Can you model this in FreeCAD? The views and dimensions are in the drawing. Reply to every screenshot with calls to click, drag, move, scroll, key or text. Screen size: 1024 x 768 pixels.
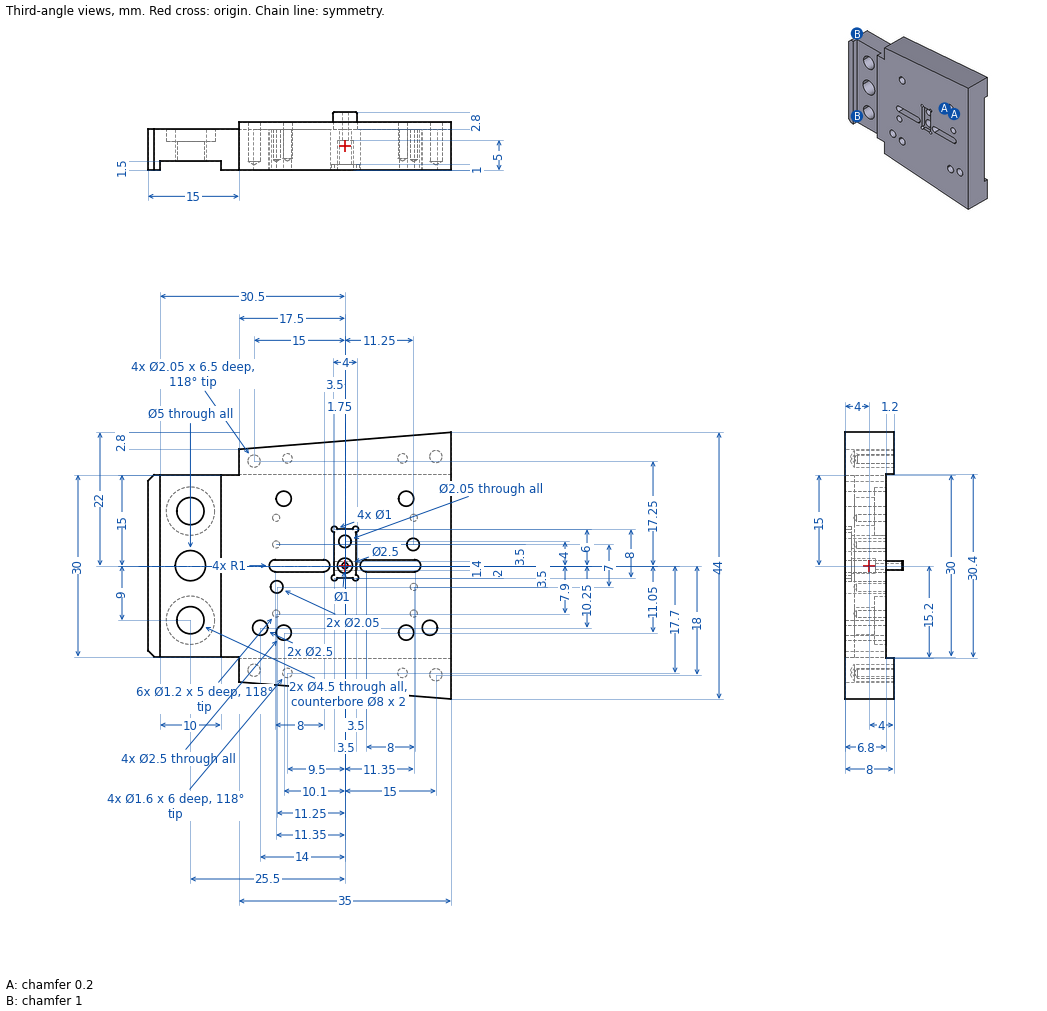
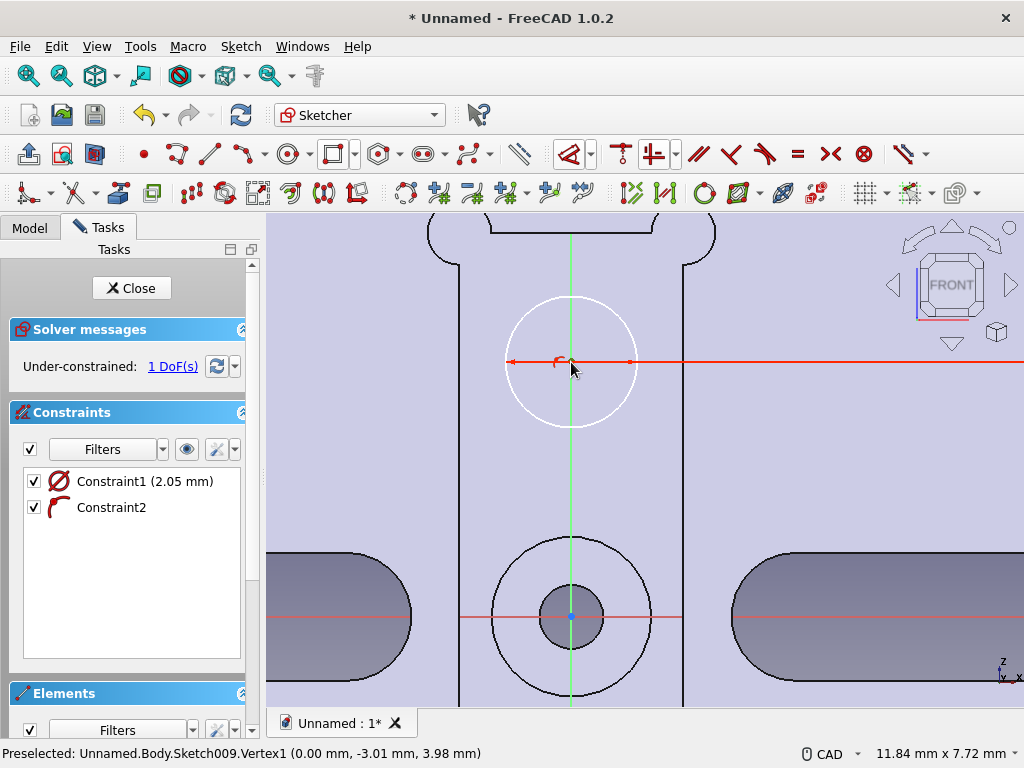
key(i)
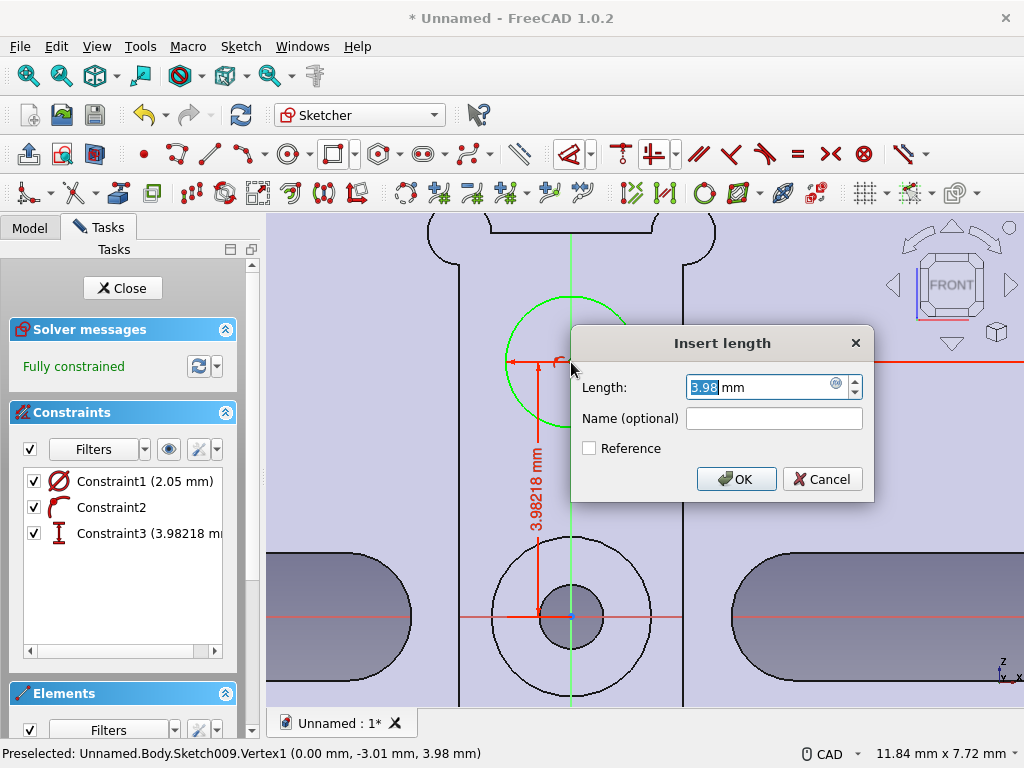
text(4)
key(Return)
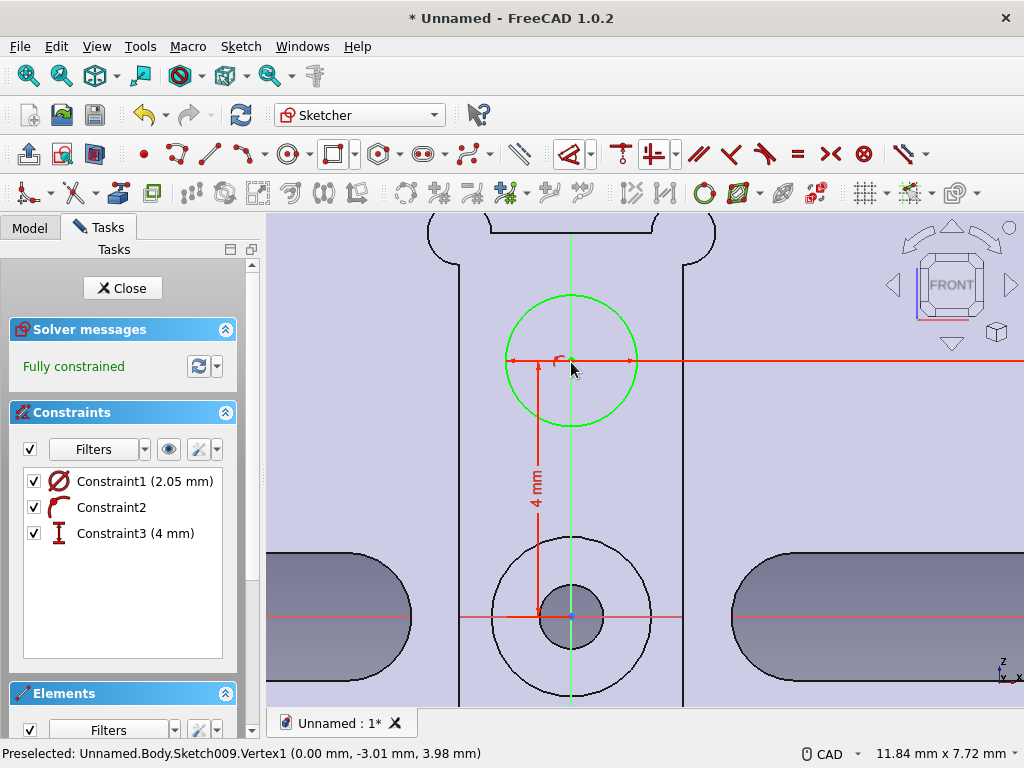
click(123, 288)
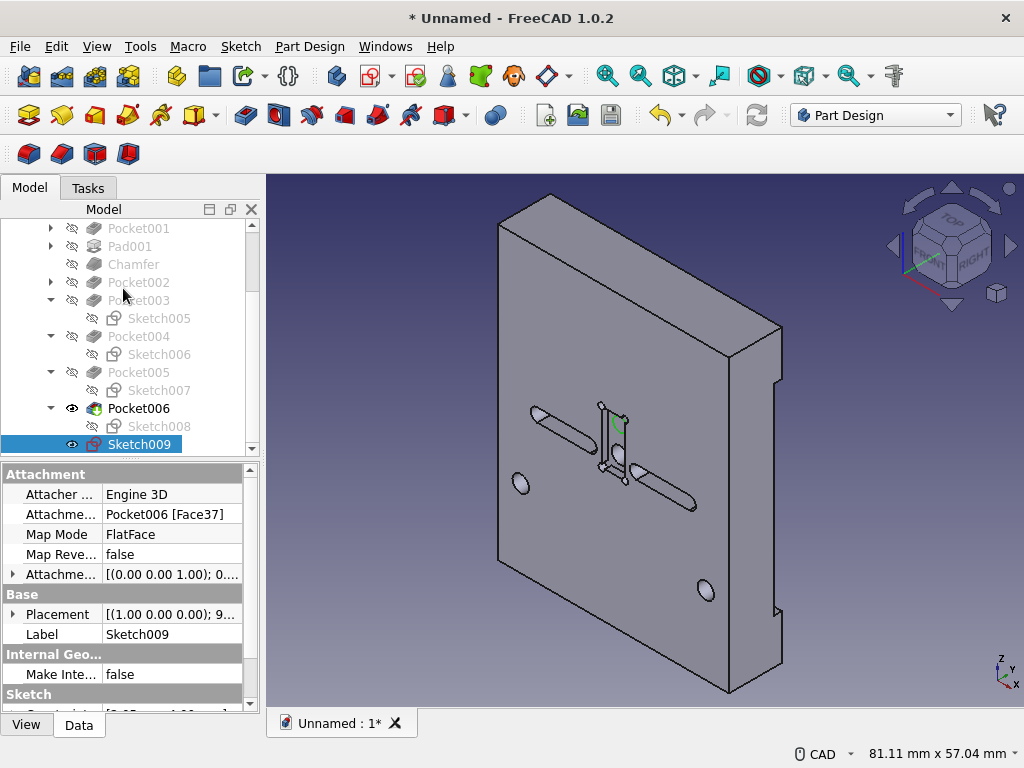
click(279, 116)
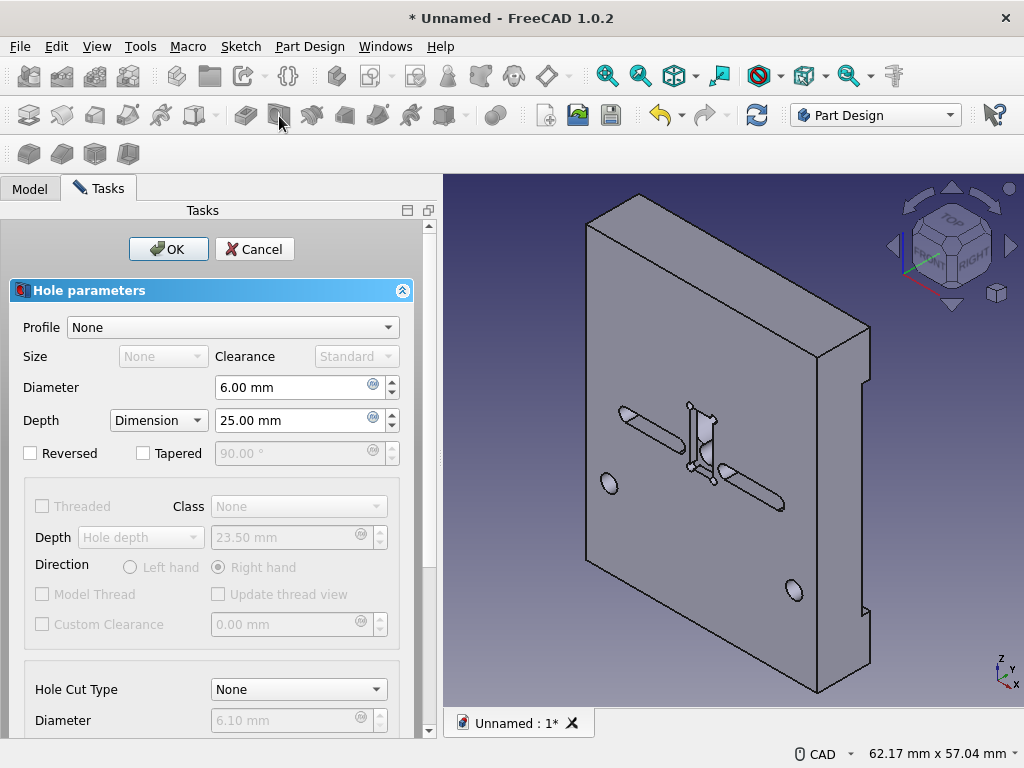
triple_click(300, 388)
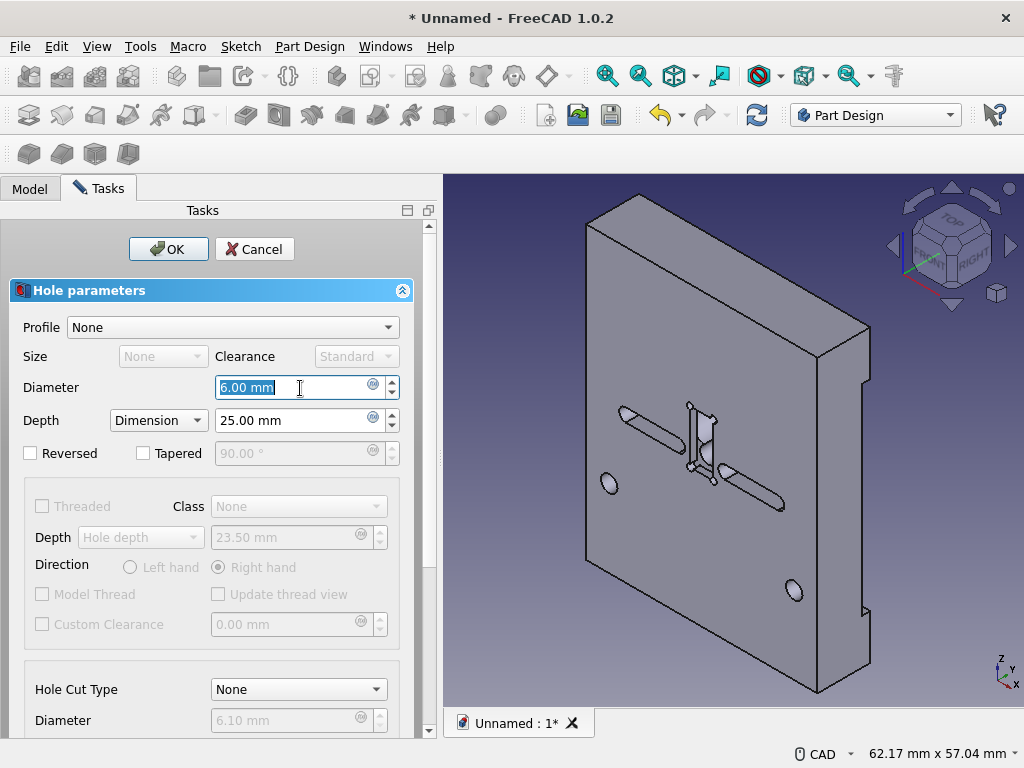
text(2.05)
key(Tab)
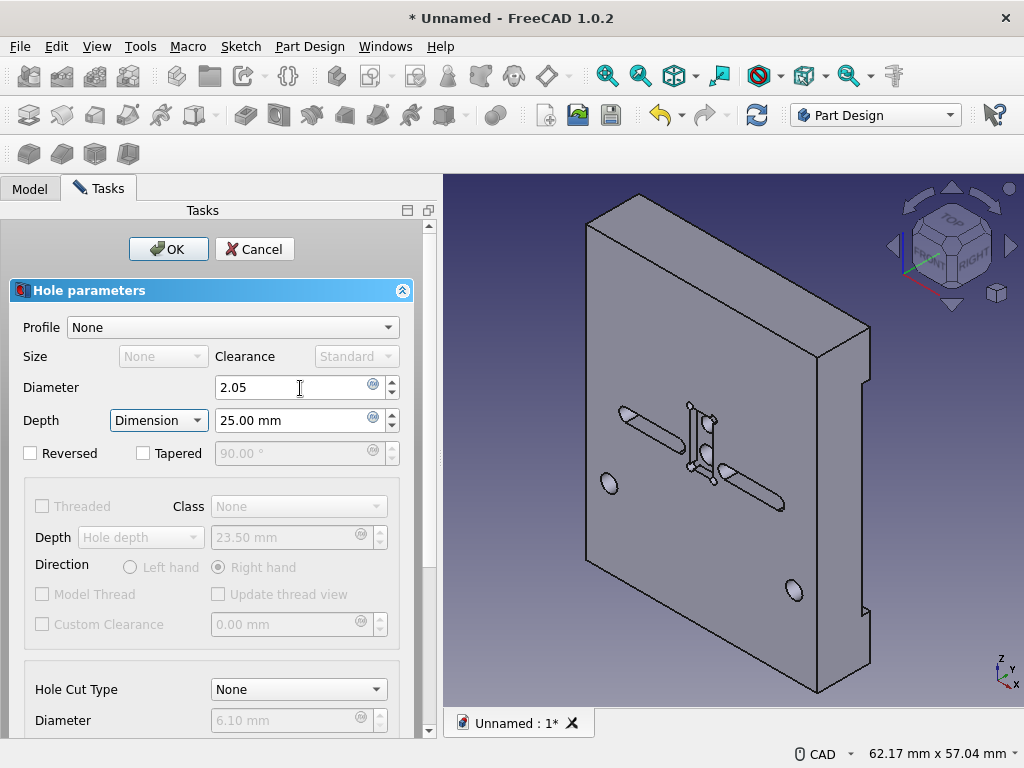
click(160, 420)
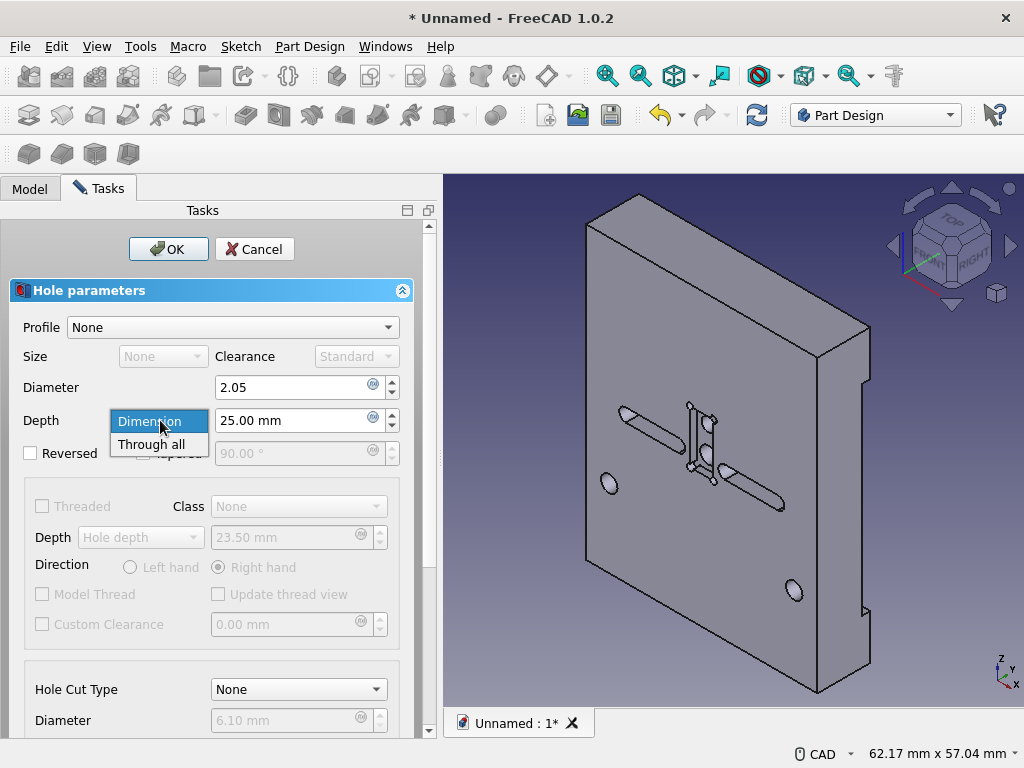
click(158, 444)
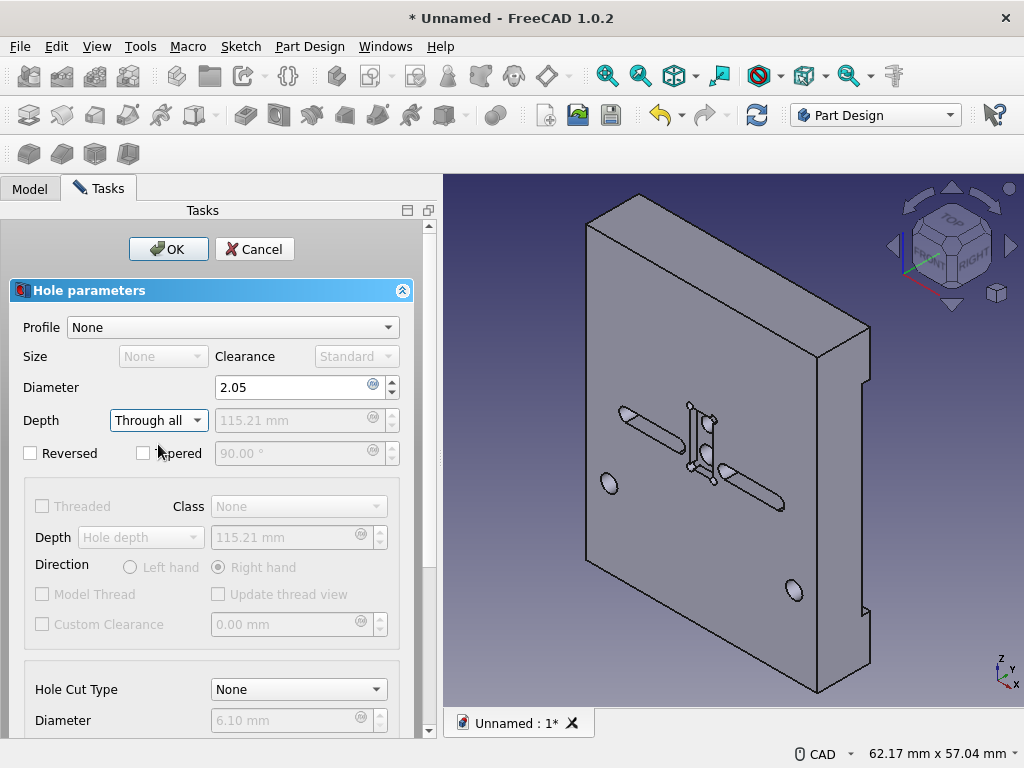
click(169, 249)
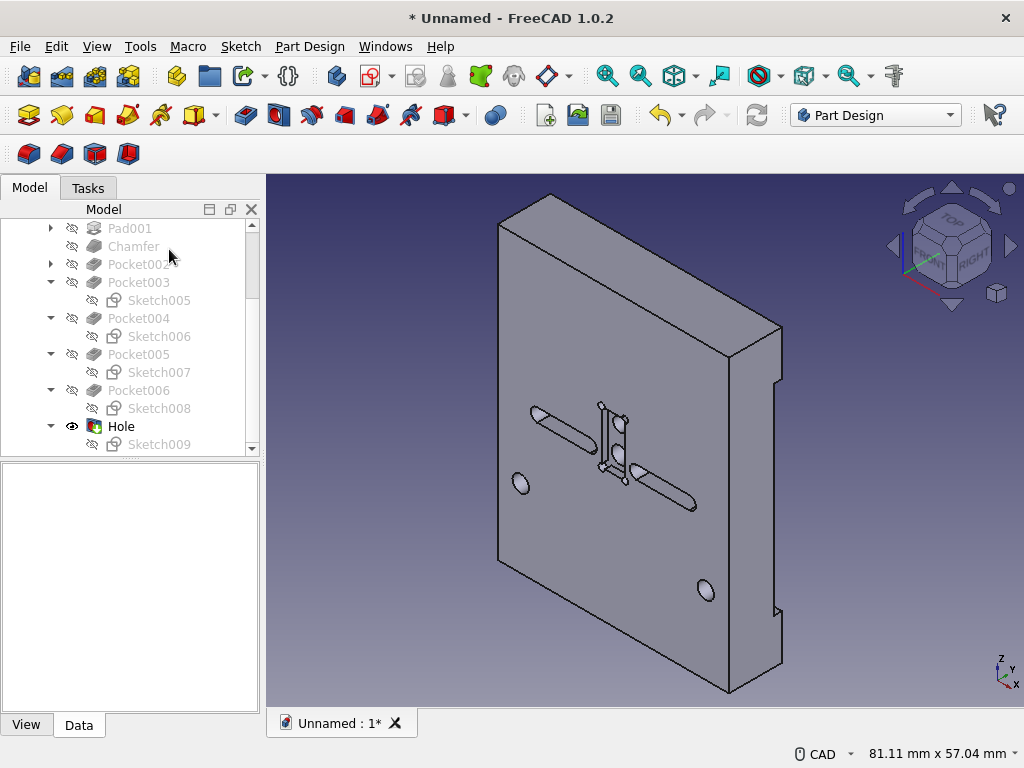
key(4)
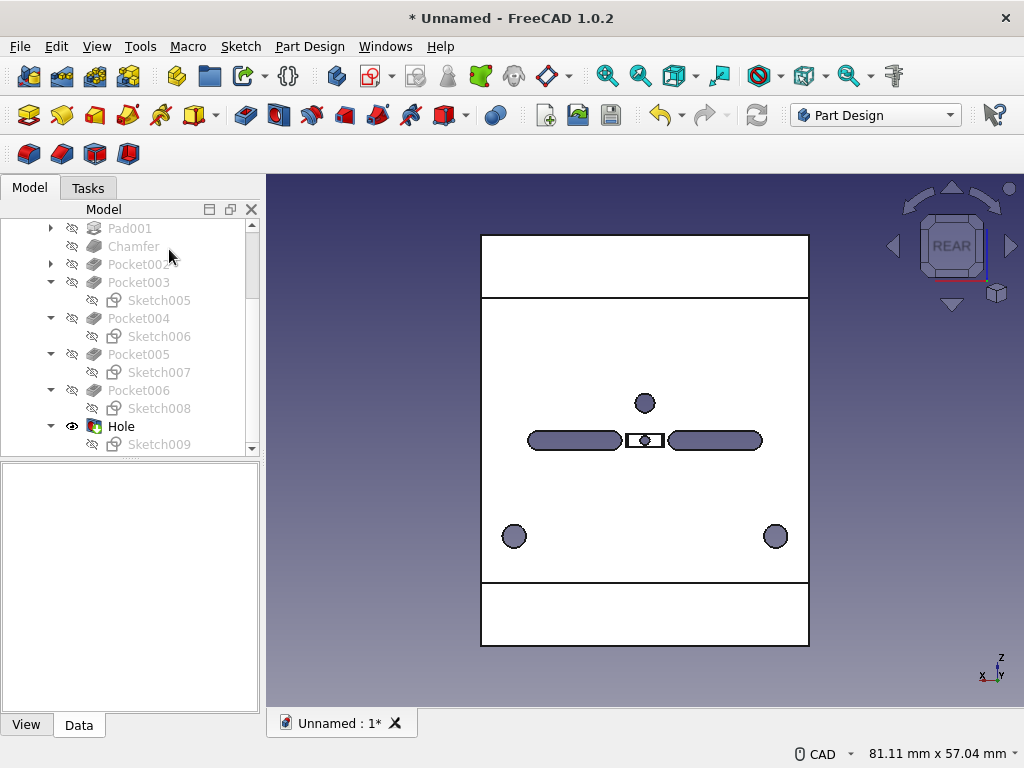
click(598, 521)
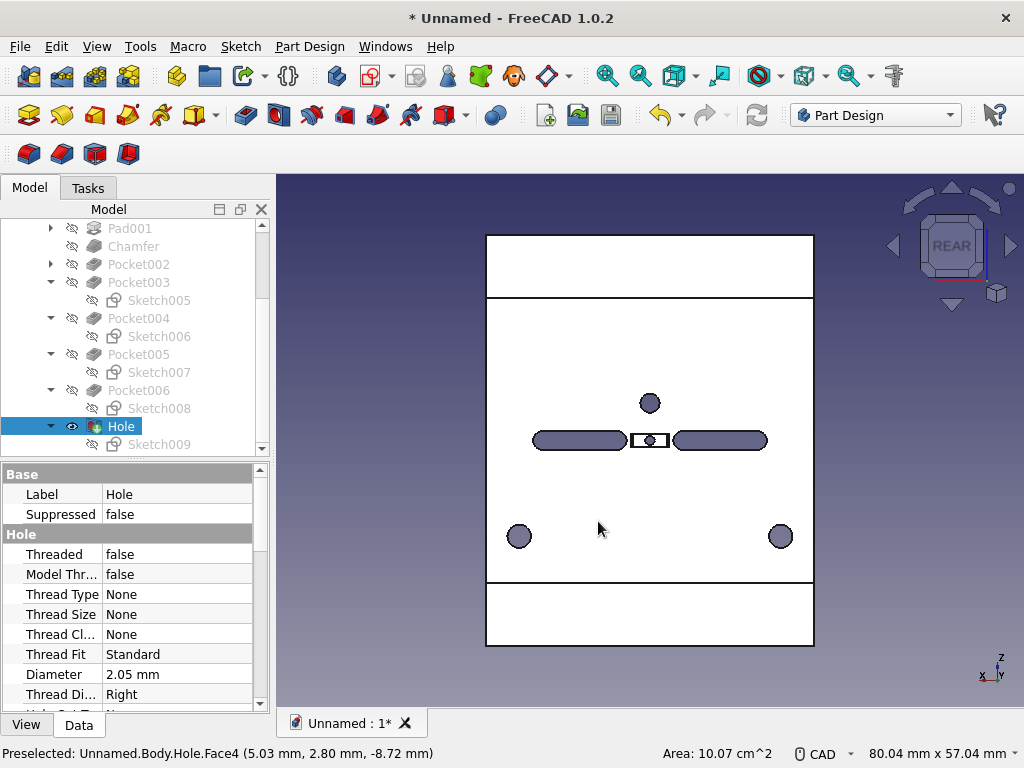
click(370, 76)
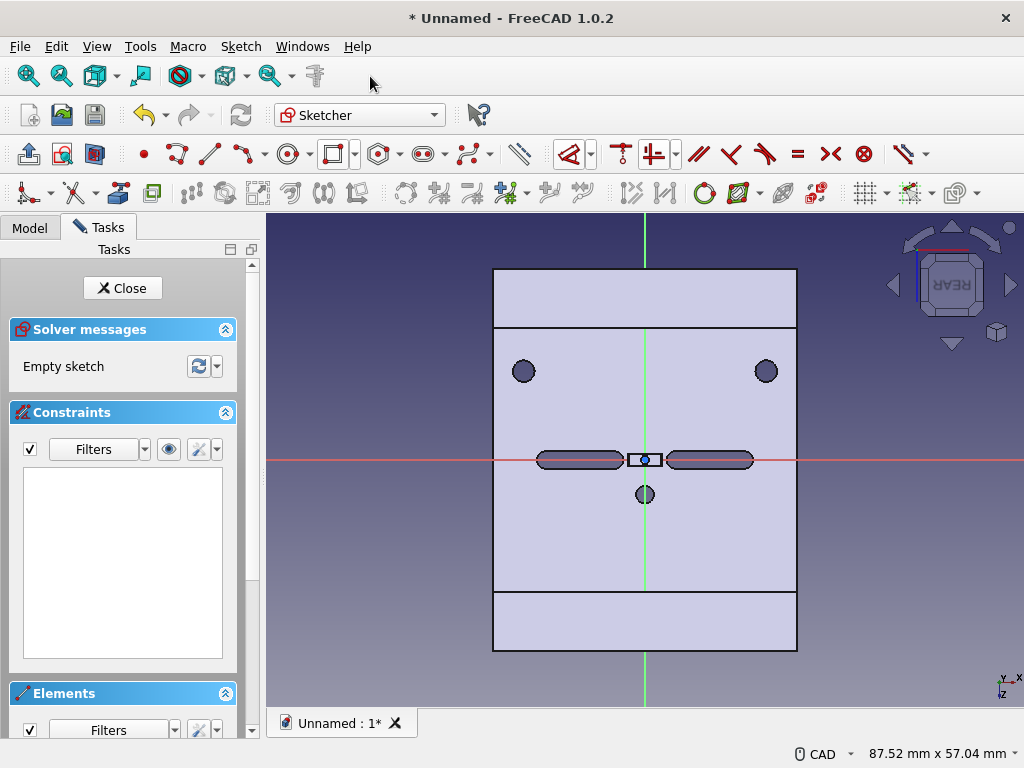
click(95, 154)